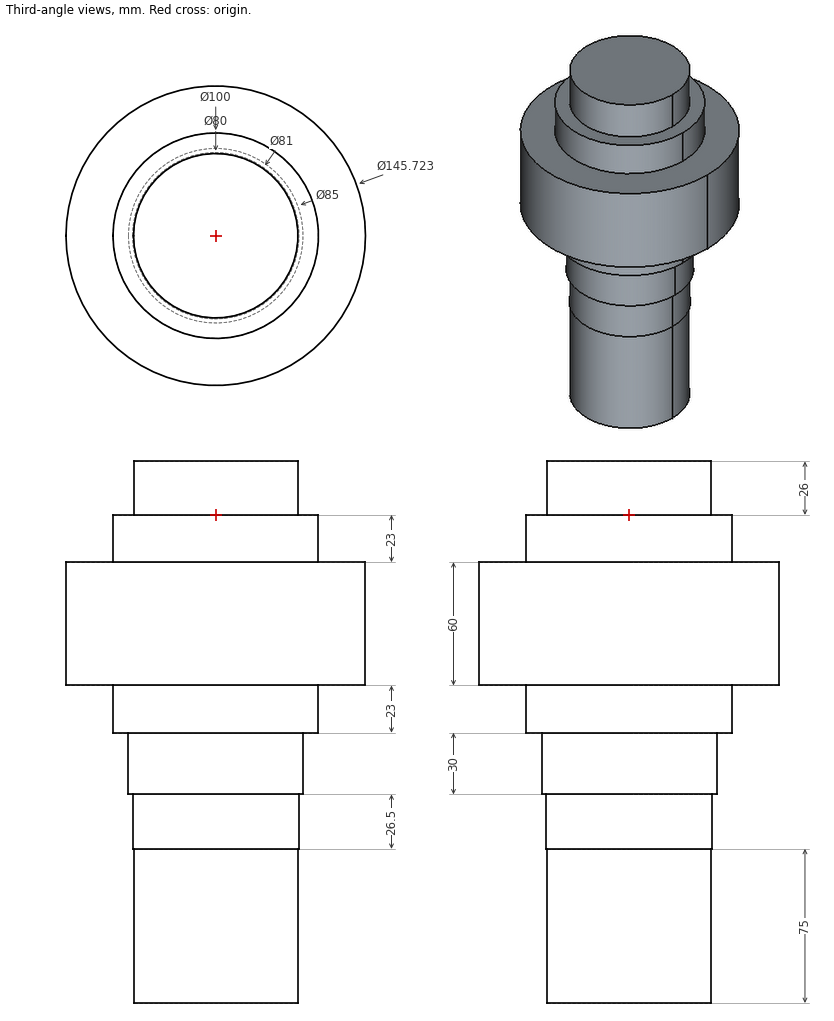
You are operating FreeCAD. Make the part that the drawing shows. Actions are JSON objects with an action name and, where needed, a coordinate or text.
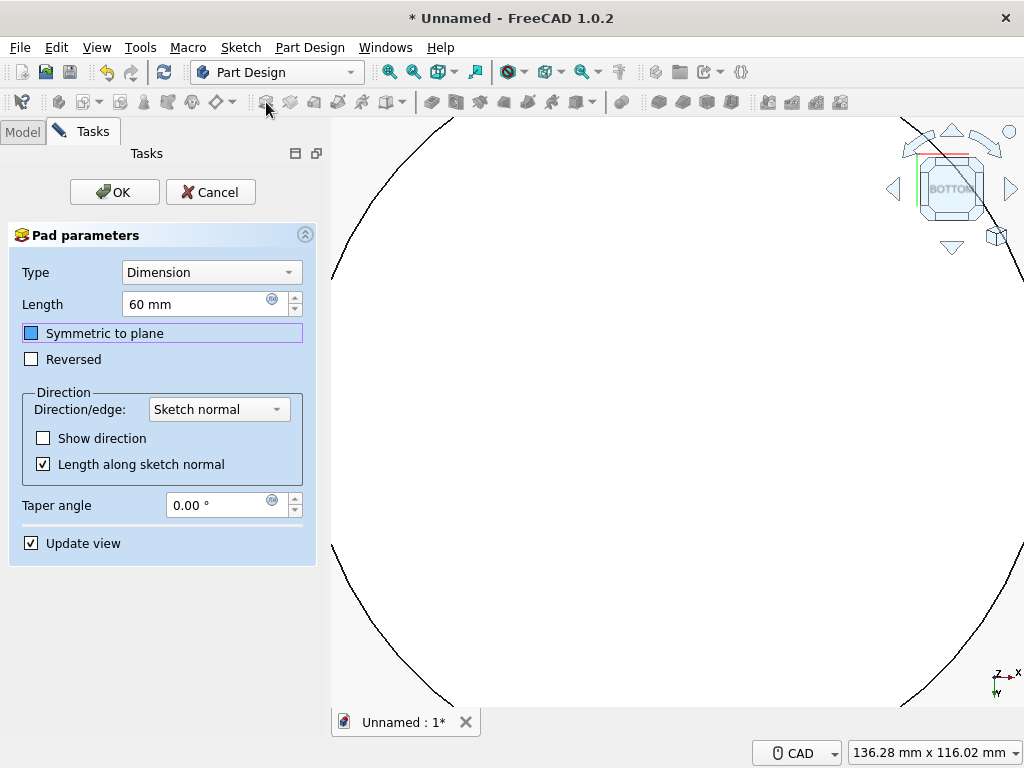
{"action": "left_click", "coordinate": [115, 192]}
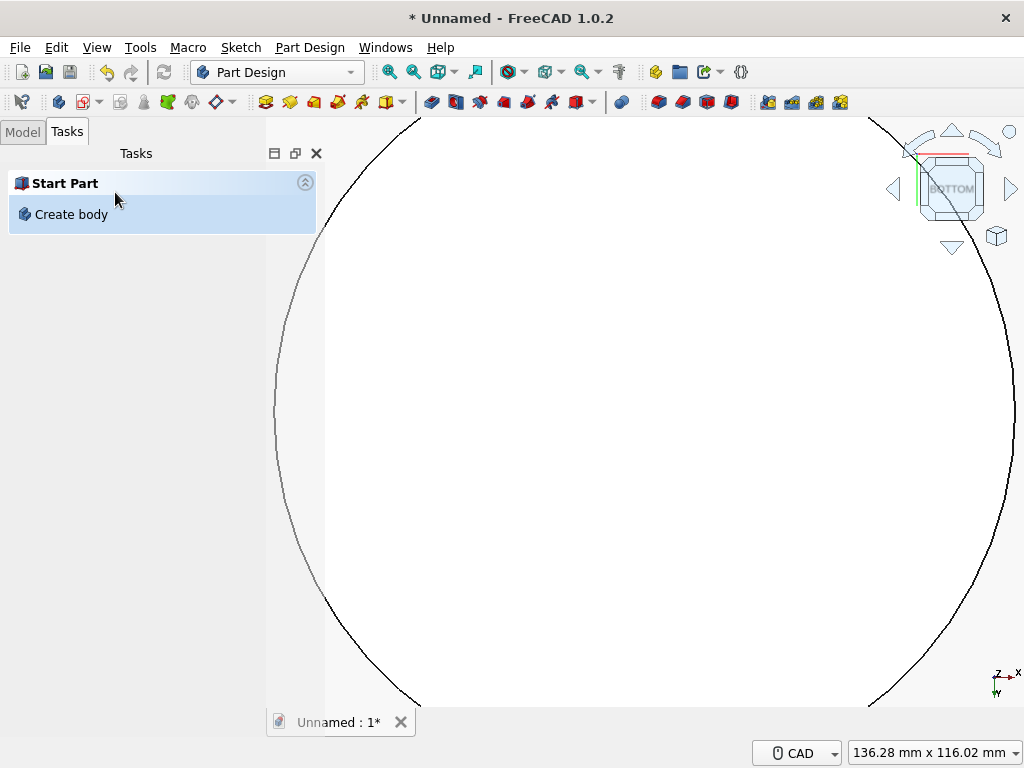
{"action": "left_click", "coordinate": [390, 72]}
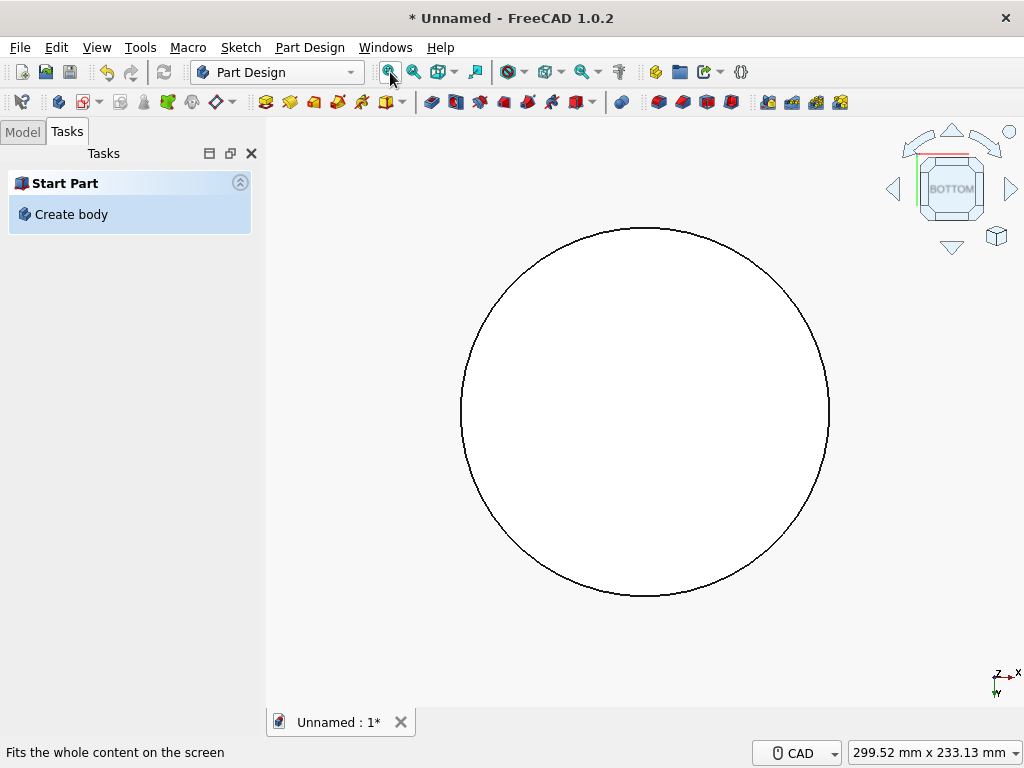
{"action": "left_click", "coordinate": [645, 411]}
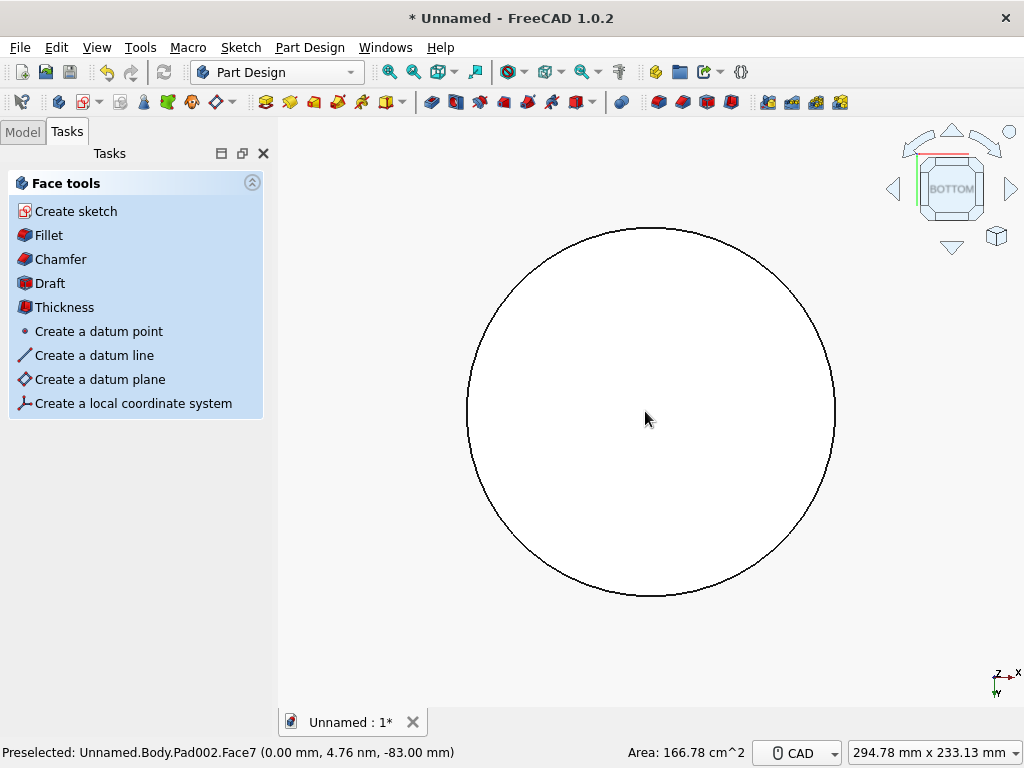
{"action": "left_click", "coordinate": [84, 102]}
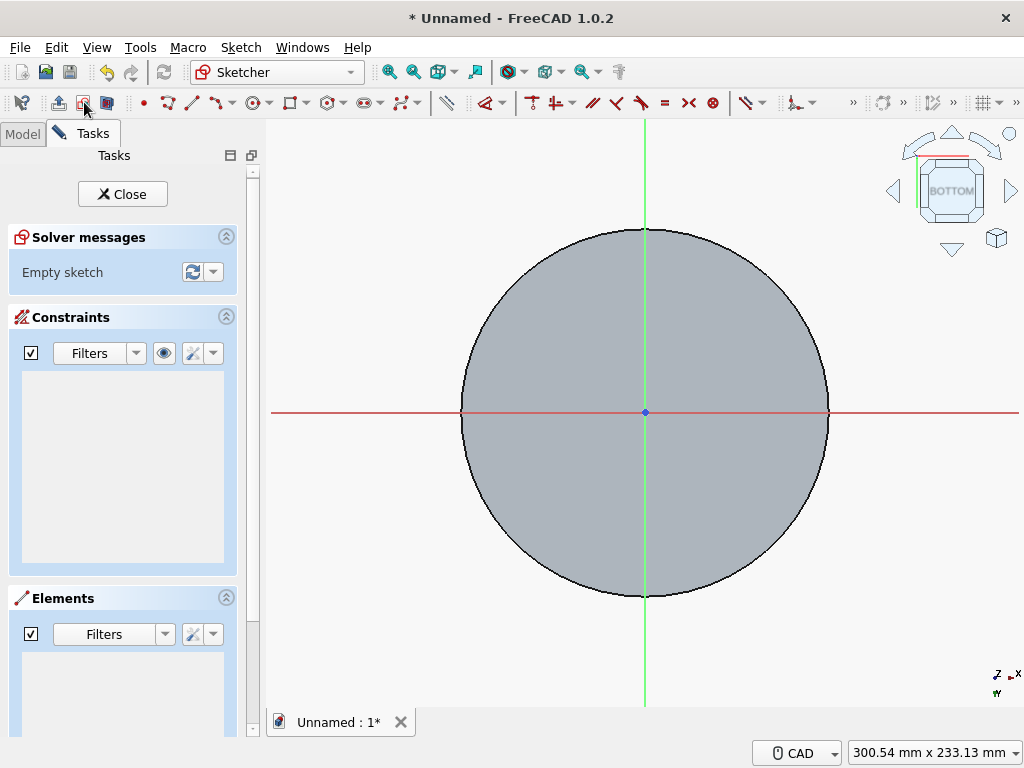
{"action": "scroll", "coordinate": [784, 413], "scroll_direction": "up", "scroll_amount": 2}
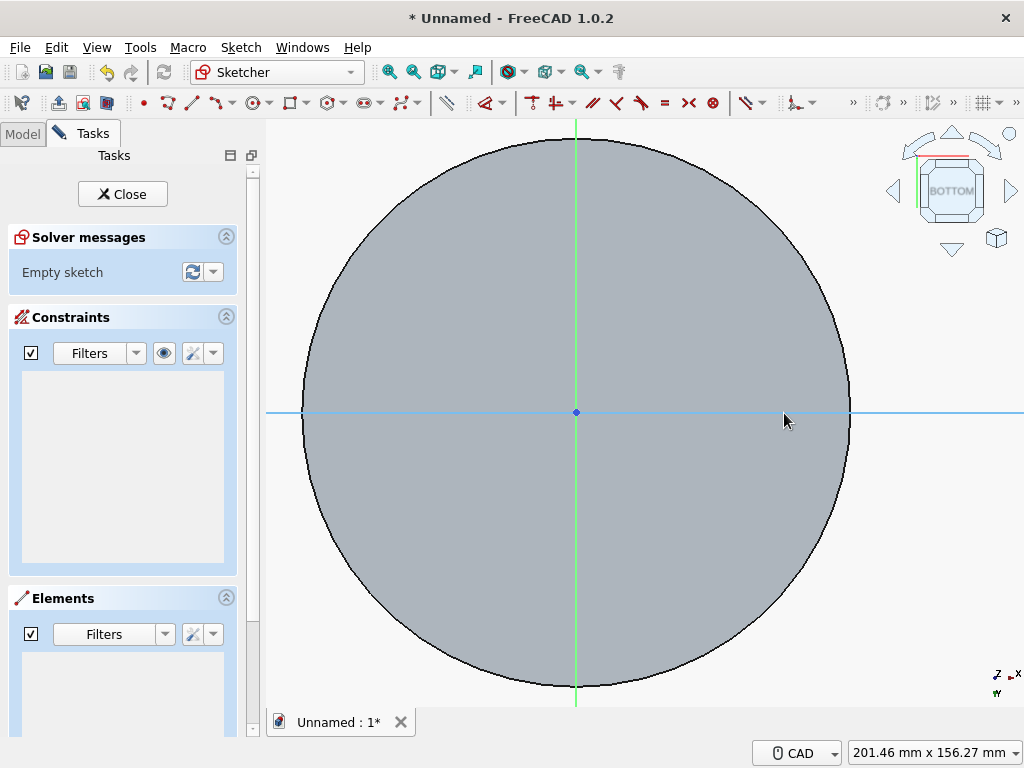
{"action": "left_click", "coordinate": [254, 104]}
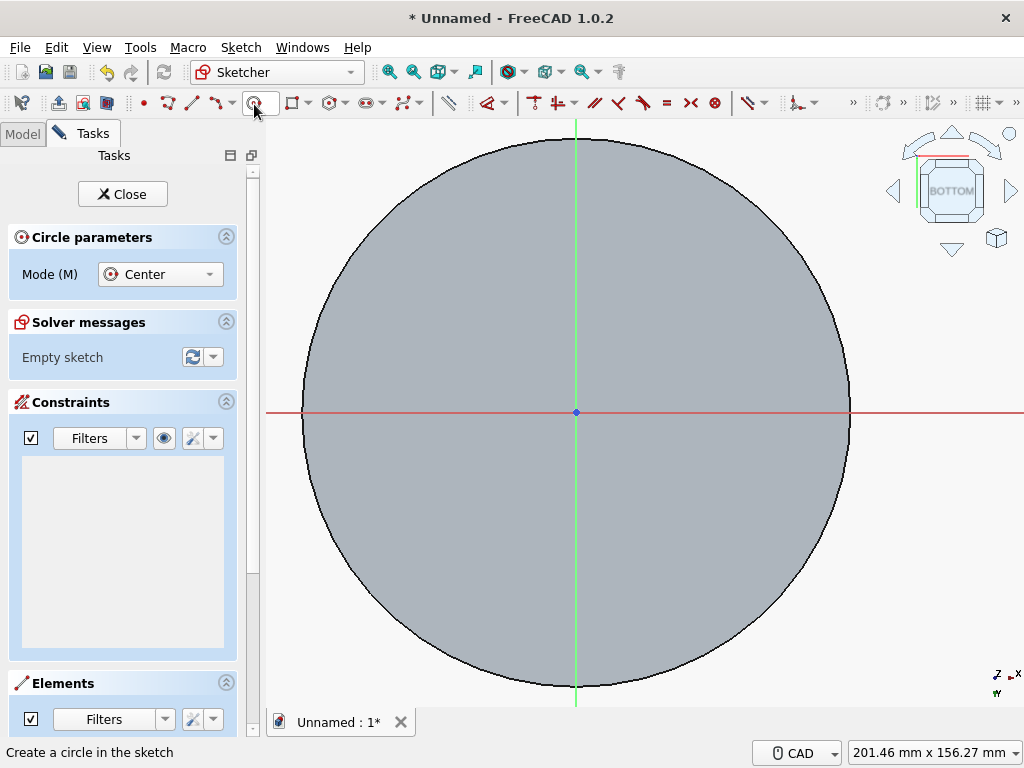
{"action": "left_click", "coordinate": [576, 413]}
{"action": "left_click", "coordinate": [709, 280]}
{"action": "key", "text": "Escape"}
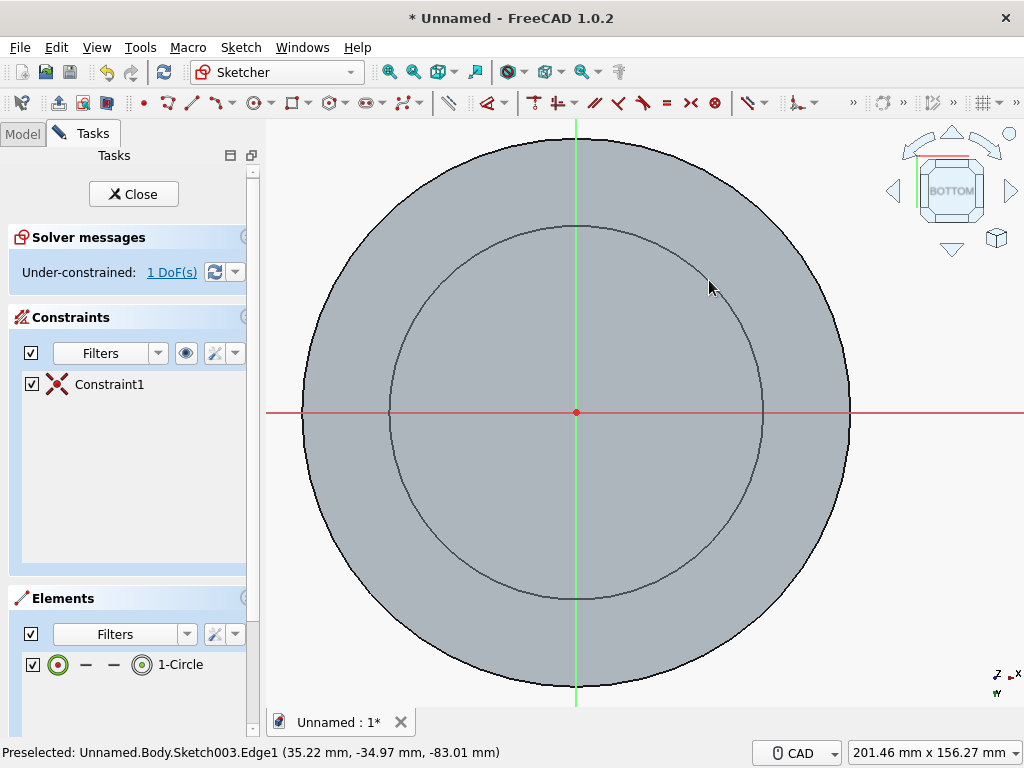
{"action": "key", "text": "d"}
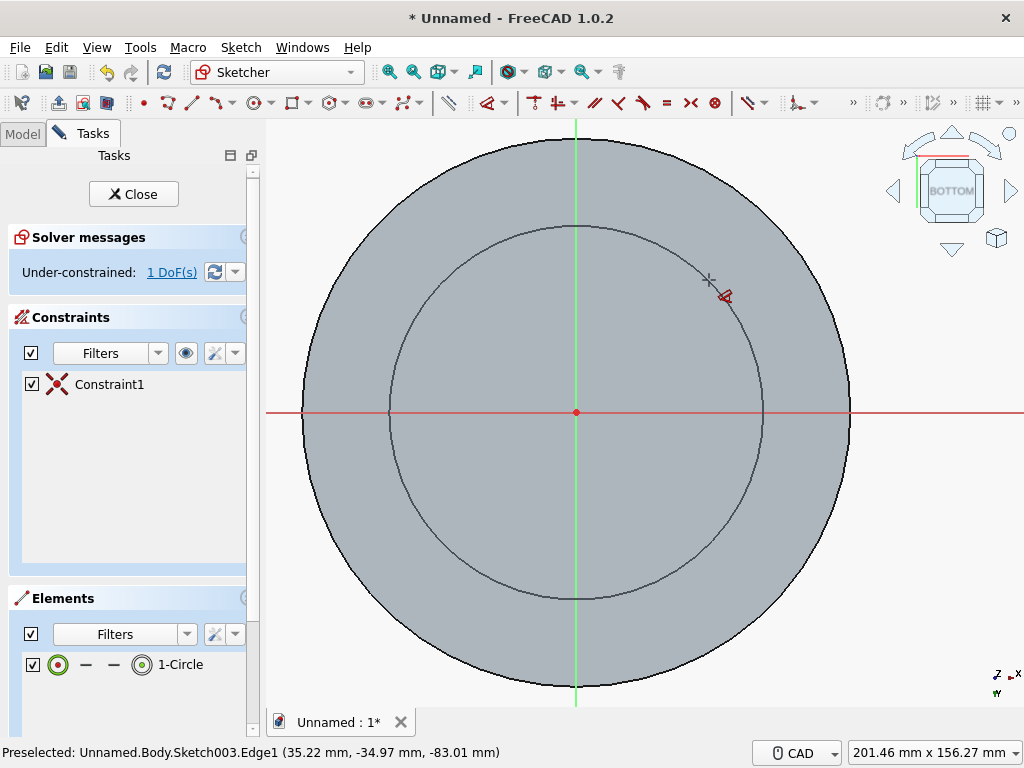
{"action": "left_click", "coordinate": [708, 280]}
{"action": "left_click", "coordinate": [731, 257]}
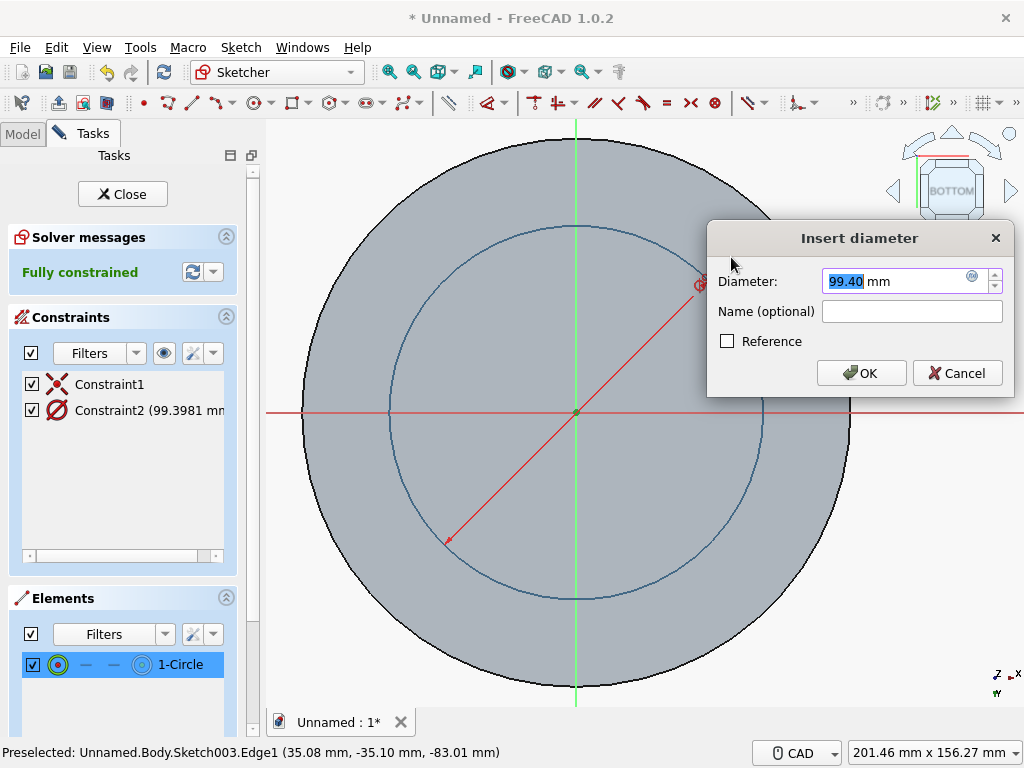
{"action": "type", "text": "100"}
{"action": "key", "text": "Return"}
{"action": "key", "text": "Escape"}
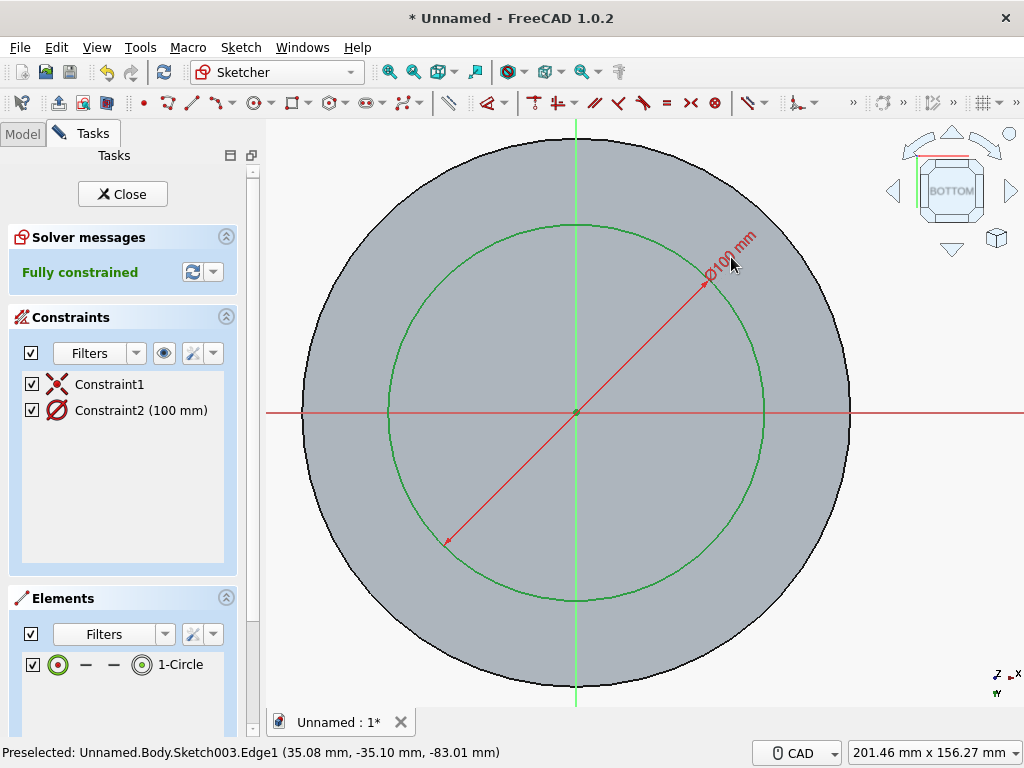
{"action": "left_click", "coordinate": [123, 194]}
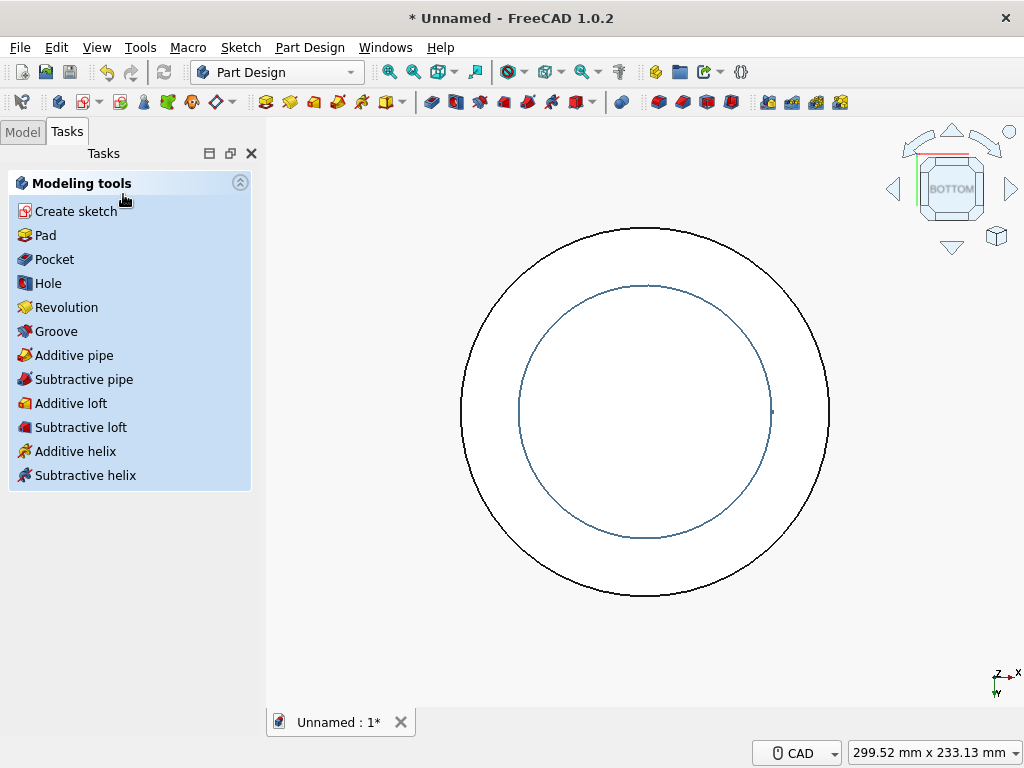
{"action": "left_click", "coordinate": [266, 102]}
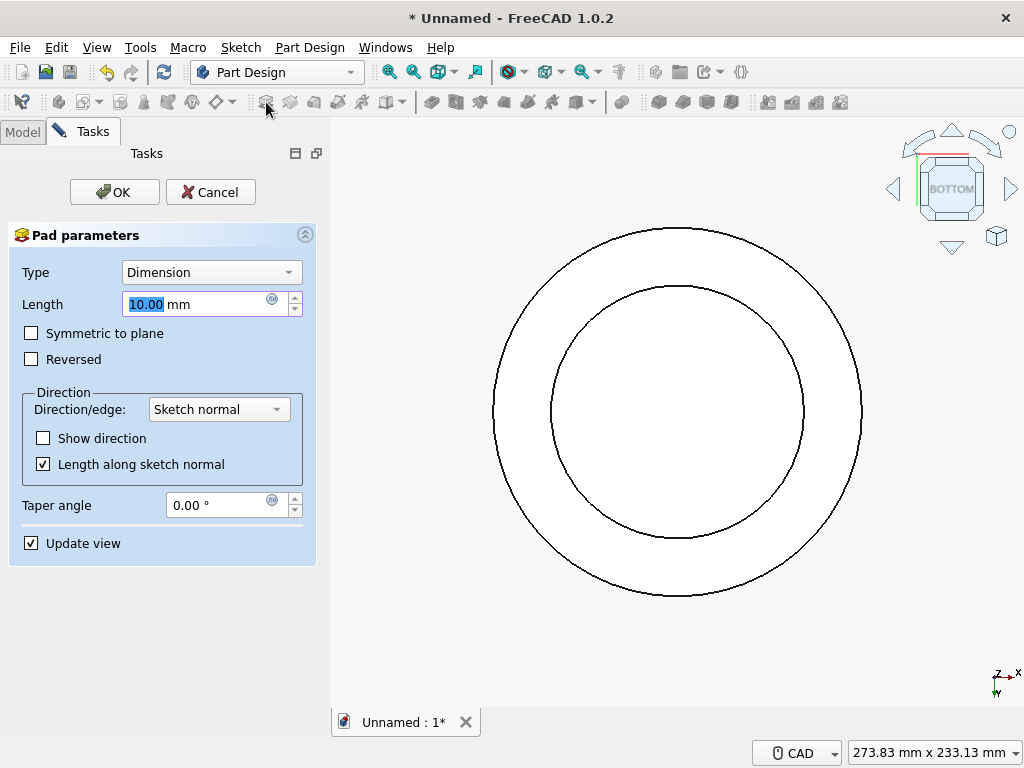
{"action": "type", "text": "23"}
{"action": "key", "text": "Tab"}